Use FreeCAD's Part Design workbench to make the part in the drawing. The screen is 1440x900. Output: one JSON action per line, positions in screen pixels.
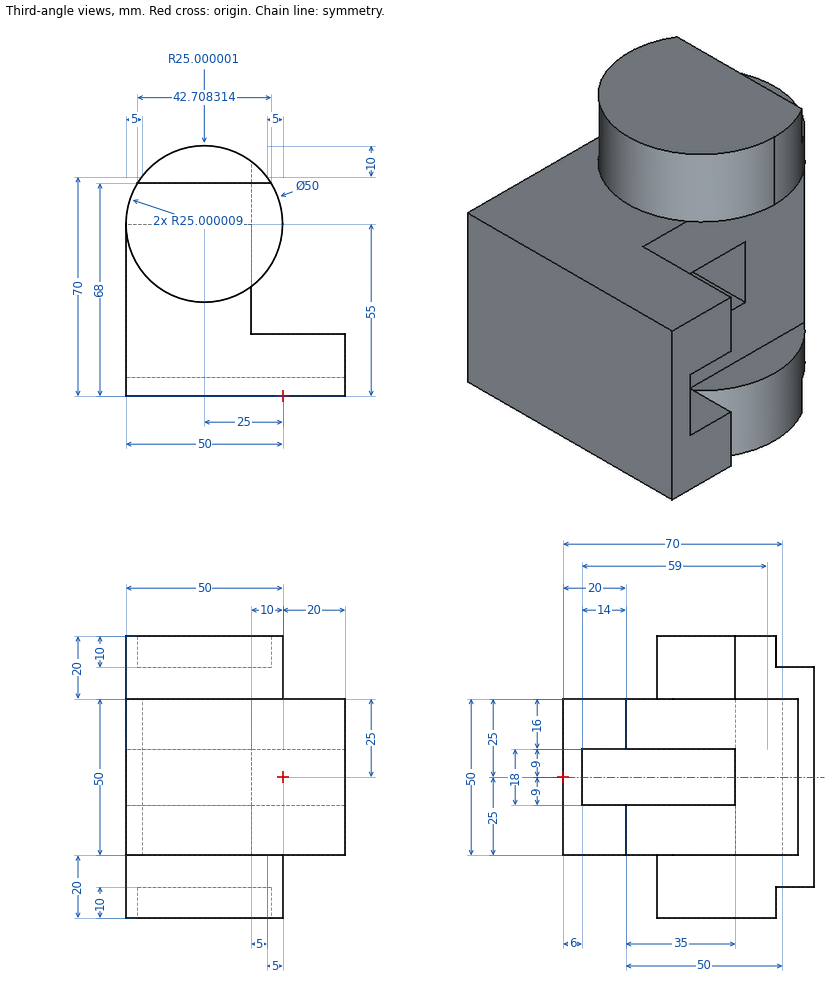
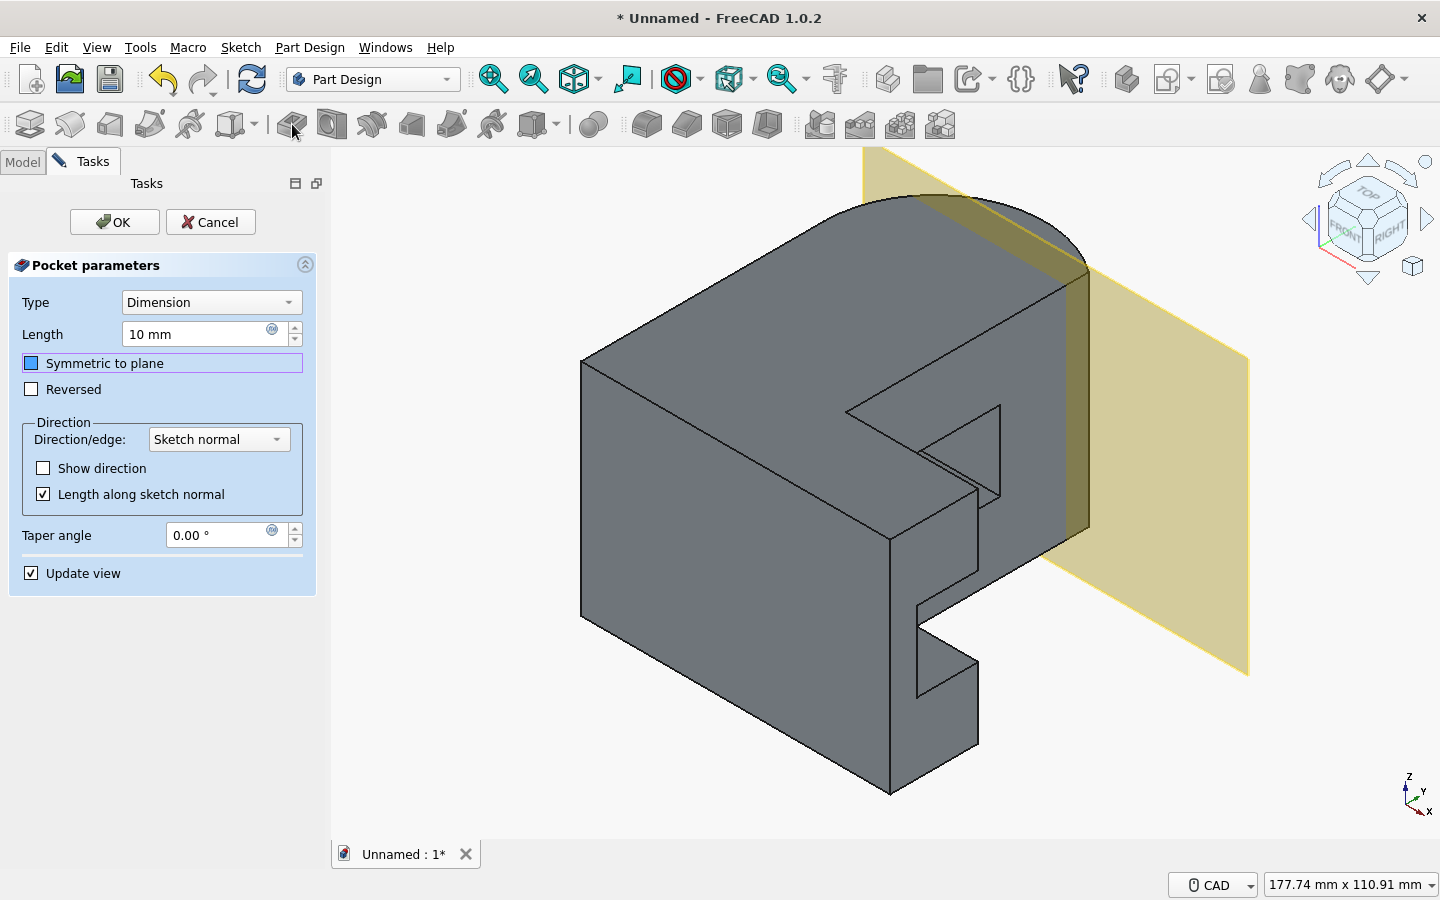
{"action": "left_click", "coordinate": [115, 222]}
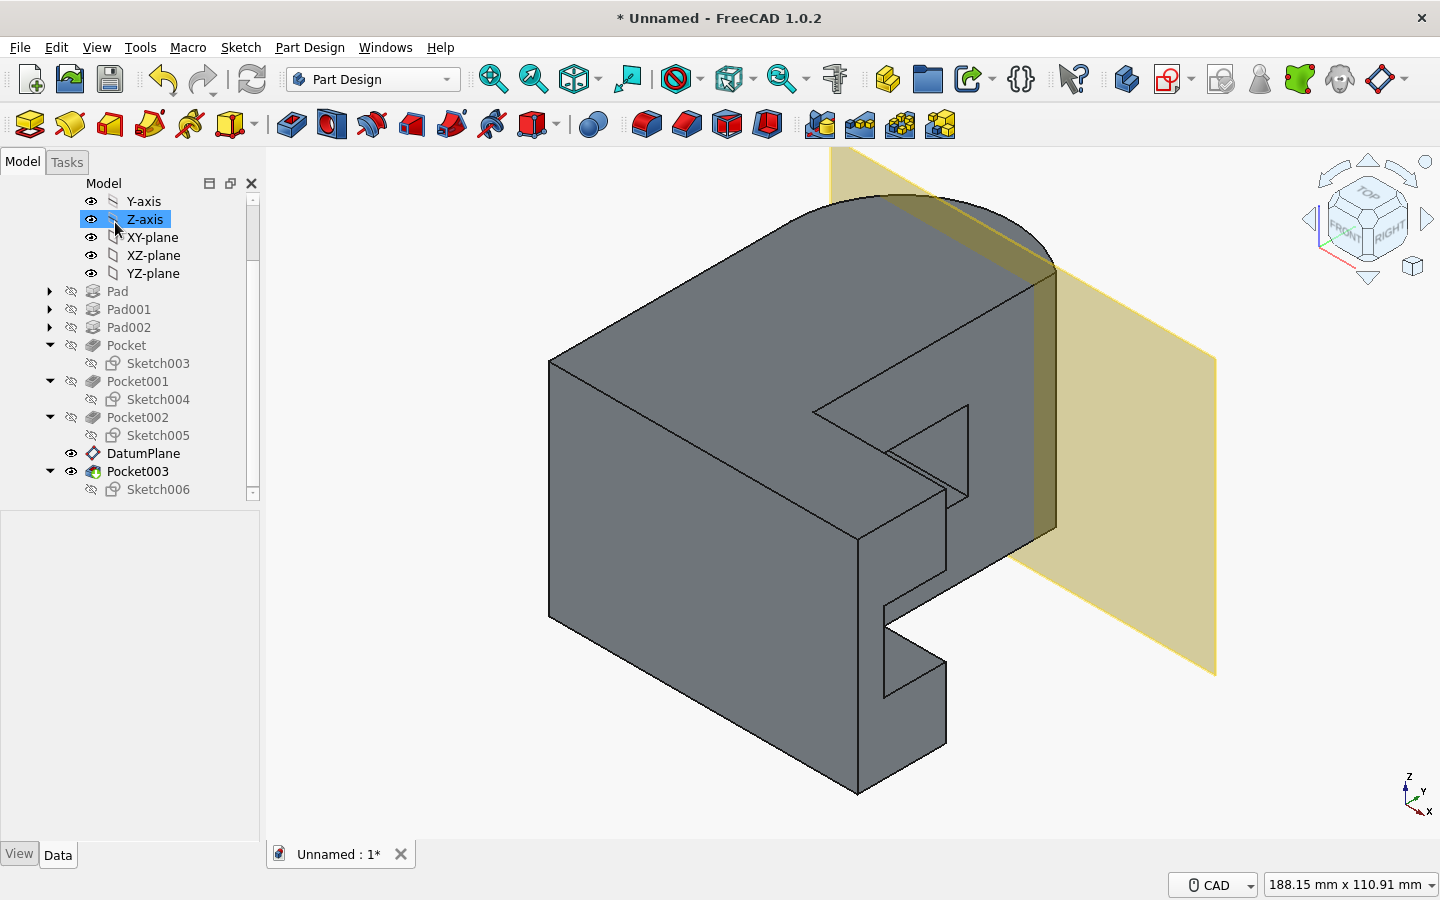
{"action": "left_click", "coordinate": [116, 453]}
{"action": "key", "text": "space"}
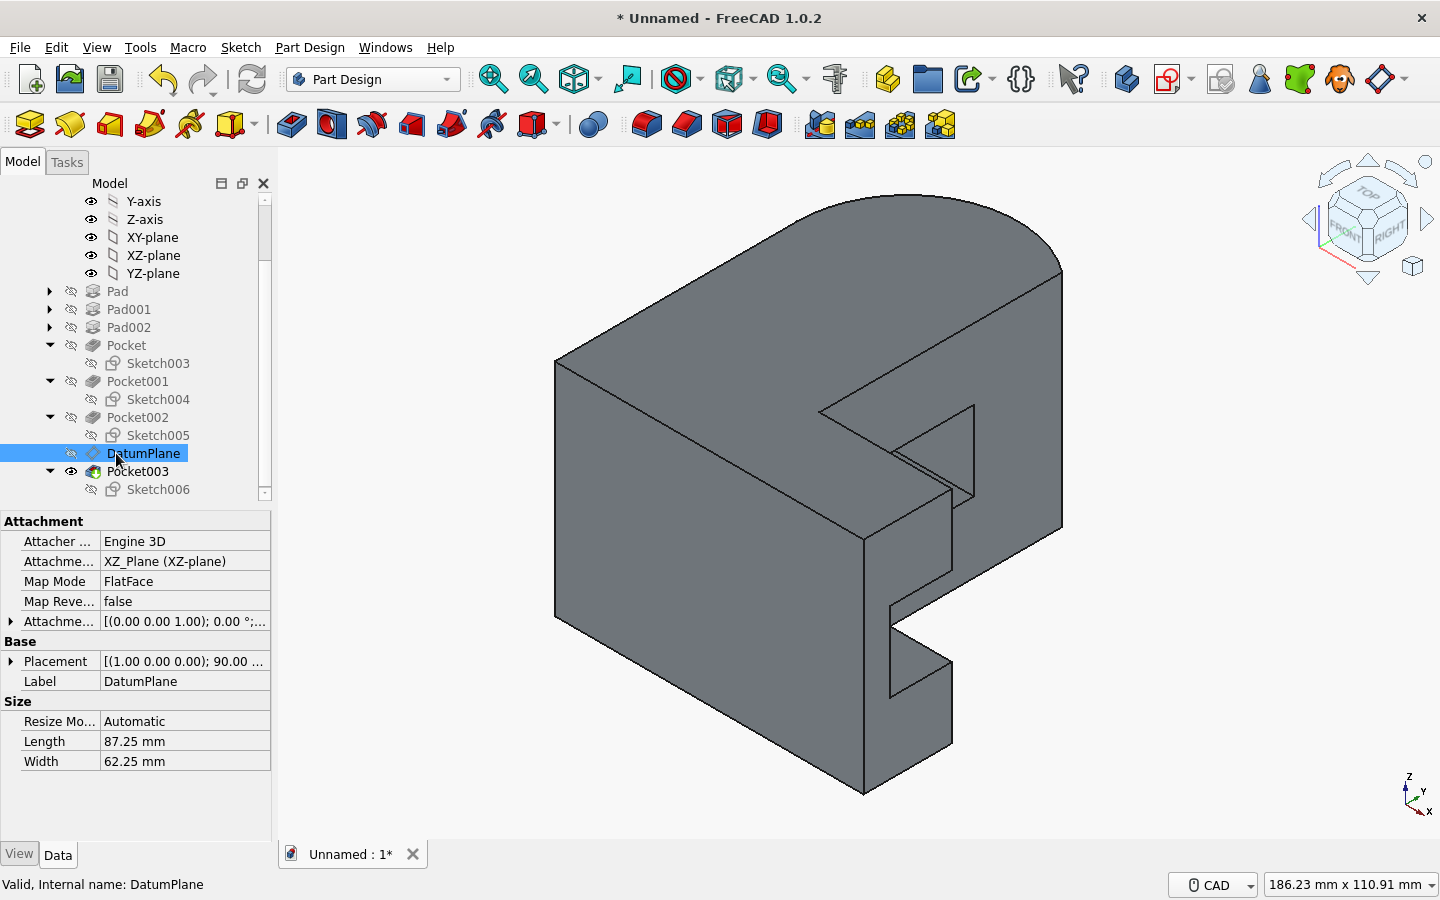
{"action": "scroll", "coordinate": [160, 341], "scroll_direction": "down", "scroll_amount": 3}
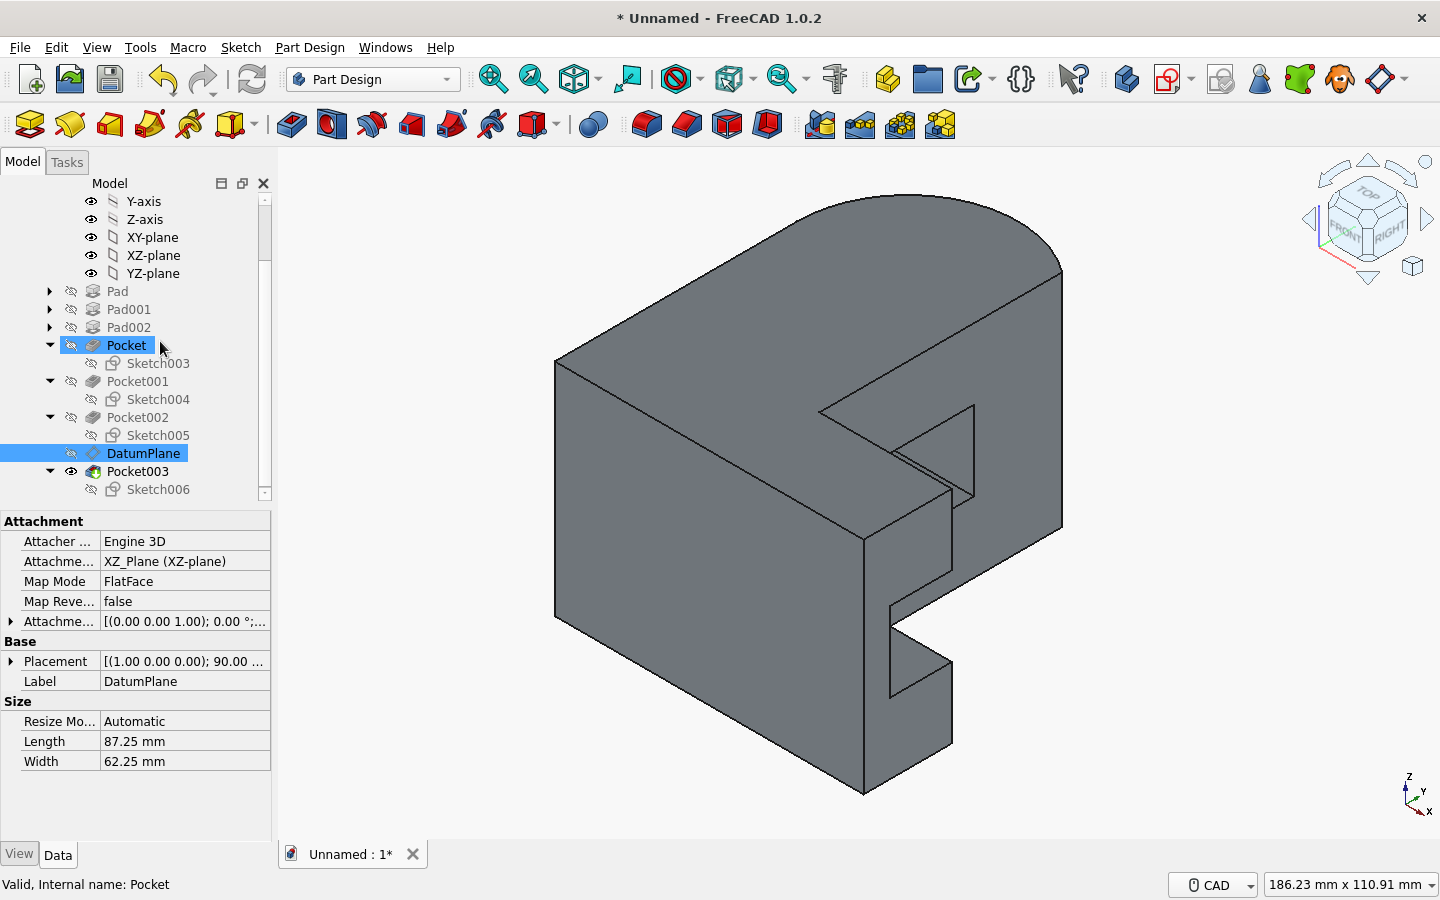
{"action": "scroll", "coordinate": [160, 341], "scroll_direction": "up", "scroll_amount": 15}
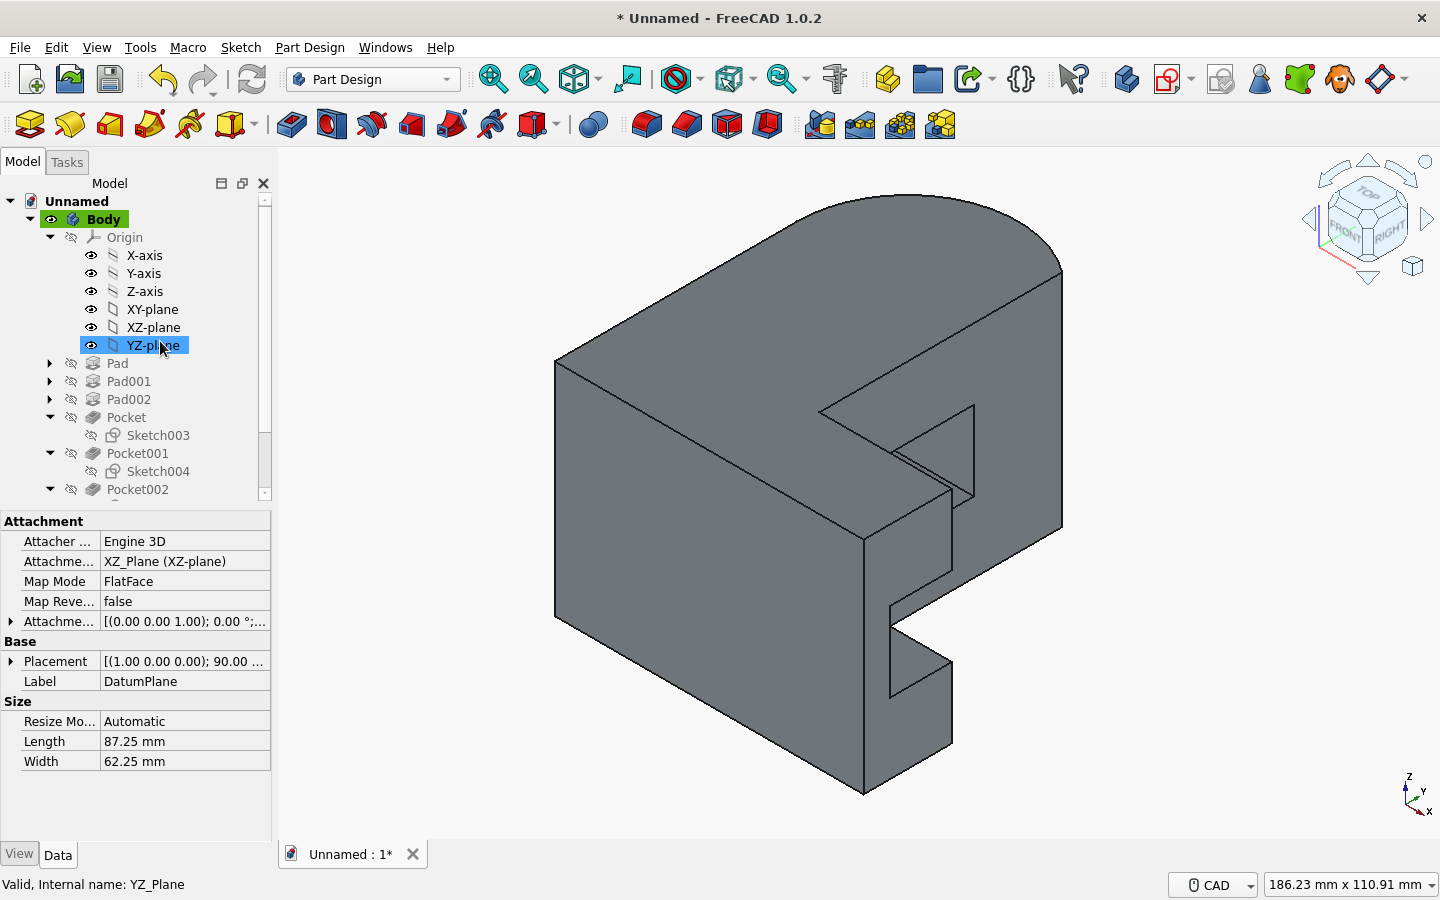
{"action": "left_click", "coordinate": [136, 309]}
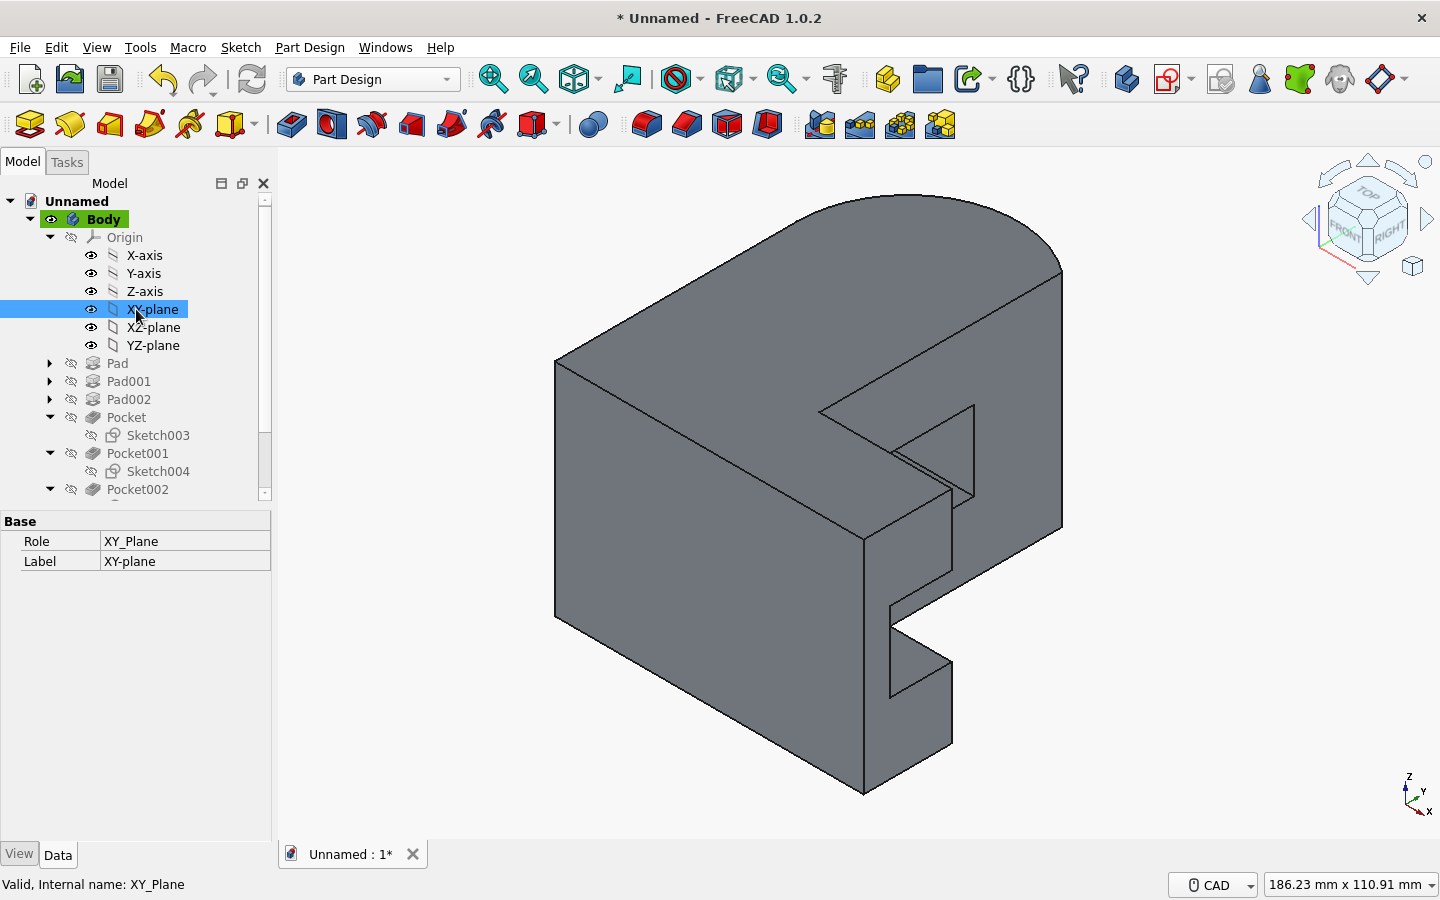
{"action": "left_click", "coordinate": [1380, 80]}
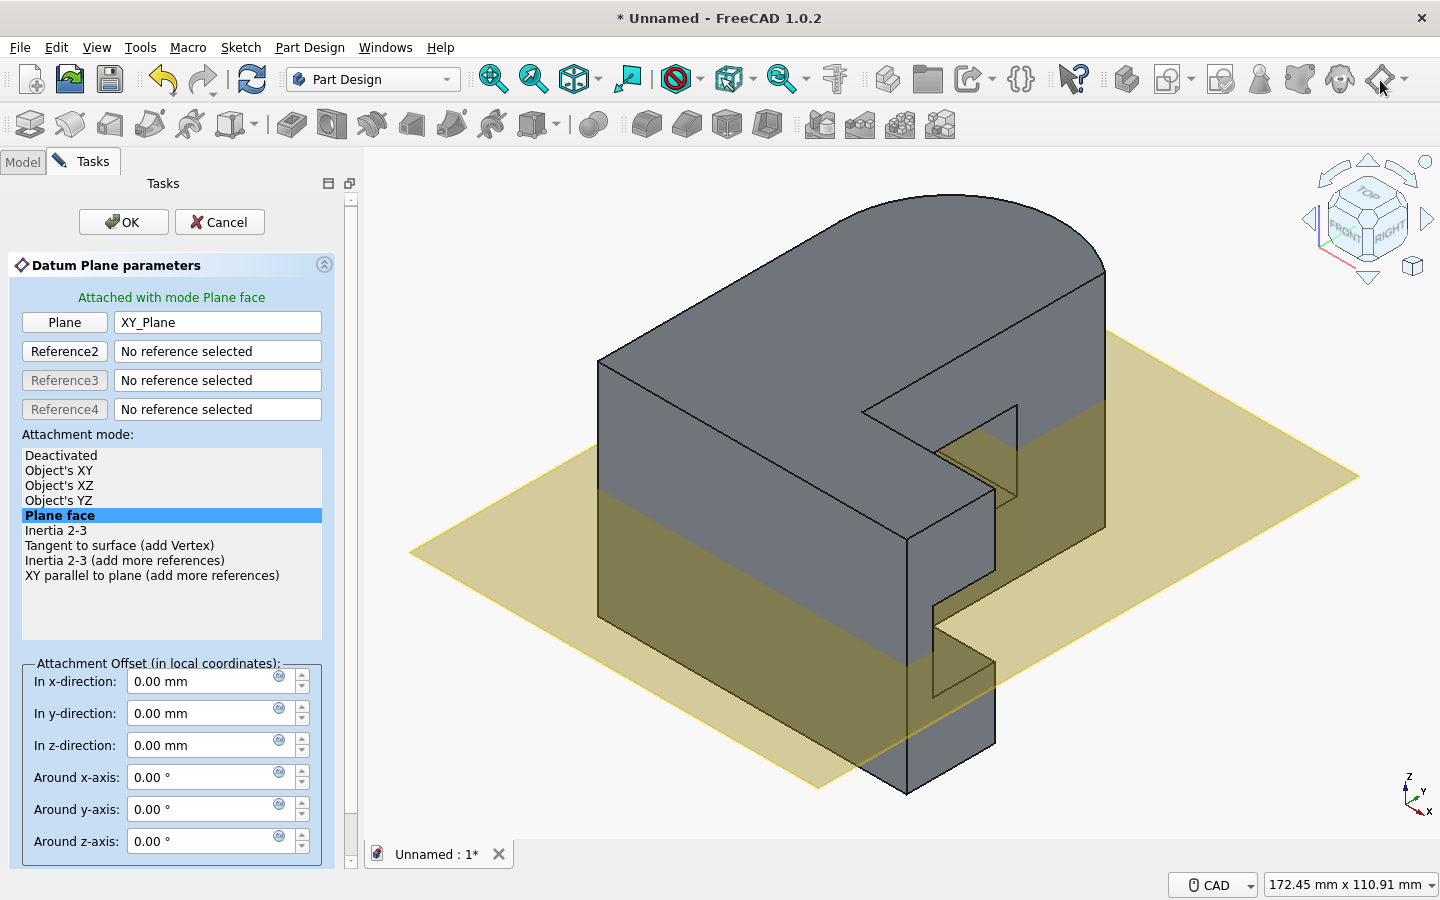
{"action": "triple_click", "coordinate": [210, 745]}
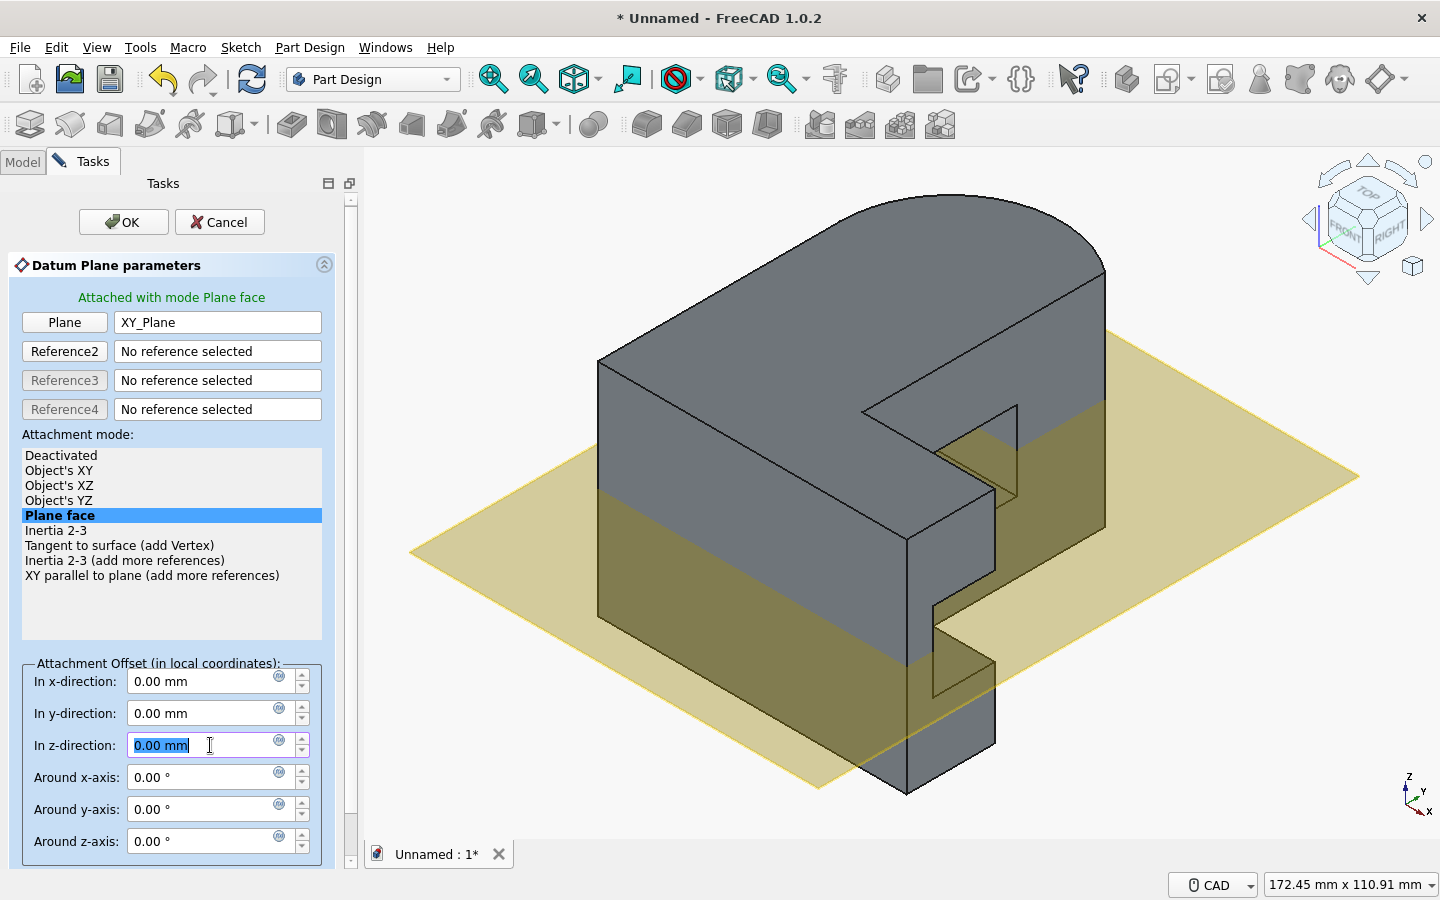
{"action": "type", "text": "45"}
{"action": "key", "text": "Tab"}